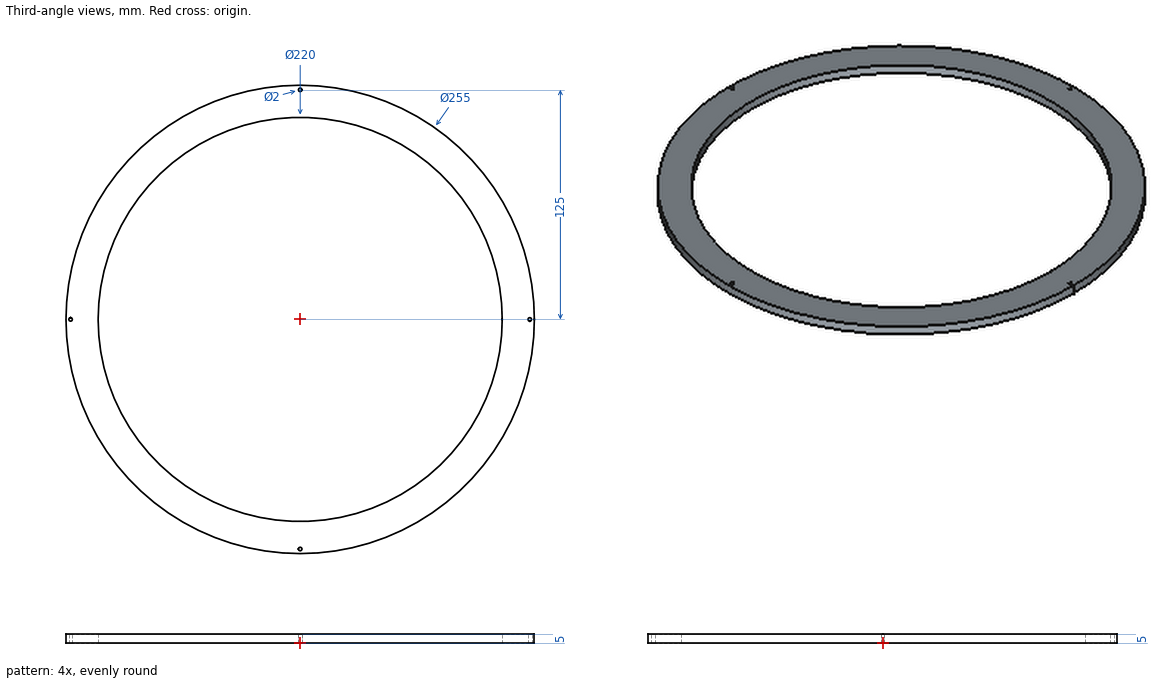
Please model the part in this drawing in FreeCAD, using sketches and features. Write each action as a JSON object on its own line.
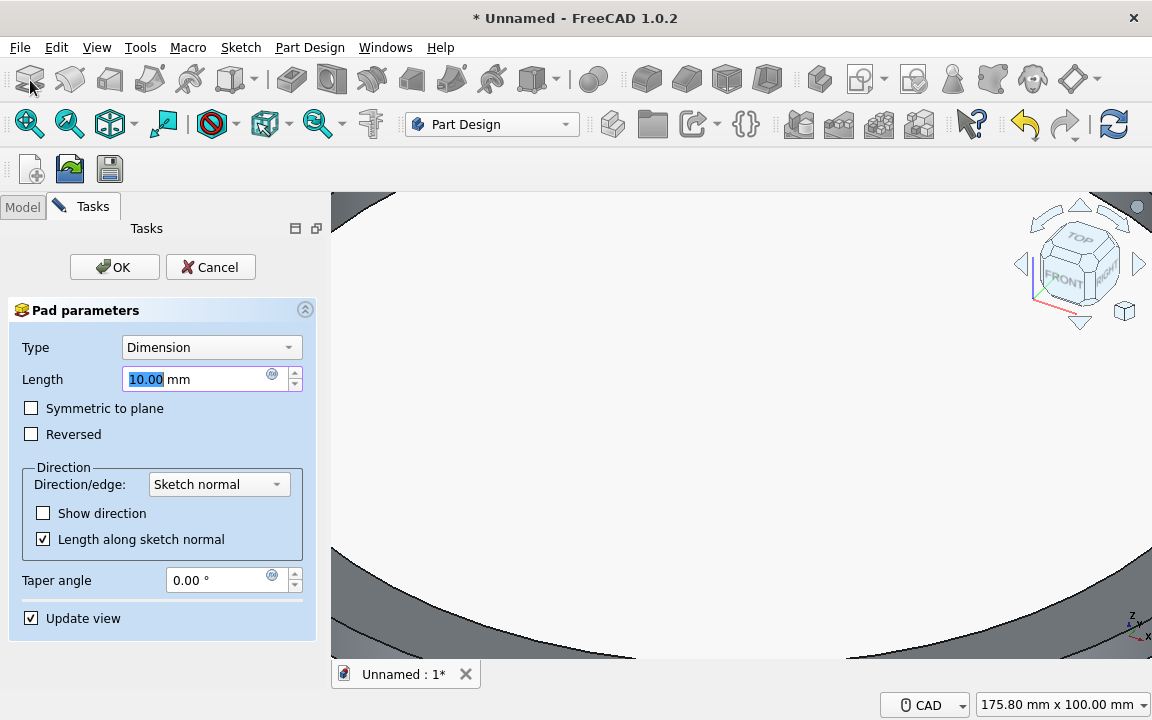
{"action": "type", "text": "5"}
{"action": "key", "text": "Tab"}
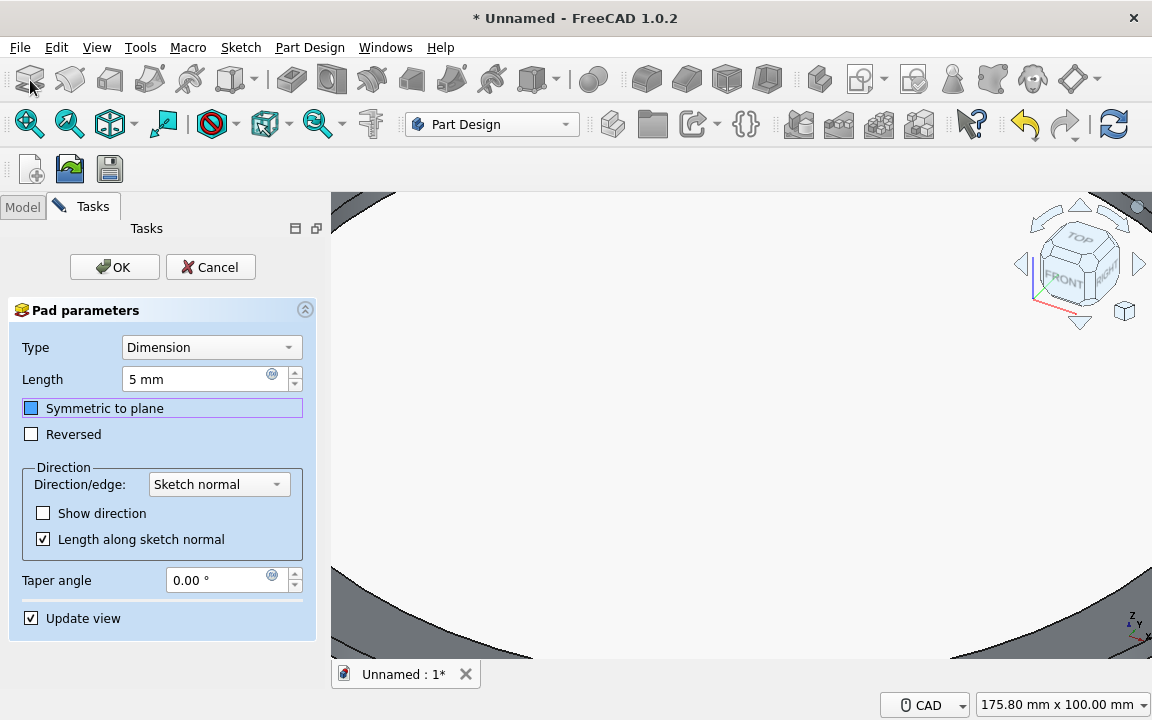
{"action": "left_click", "coordinate": [115, 267]}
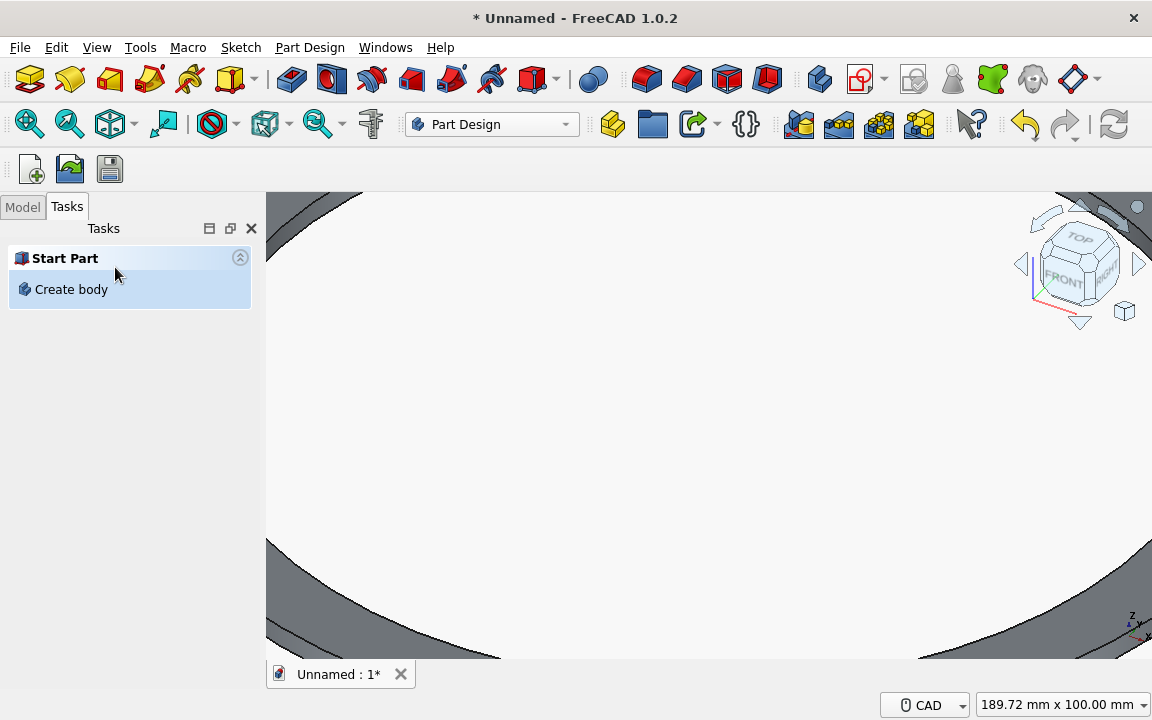
{"action": "left_click", "coordinate": [30, 124]}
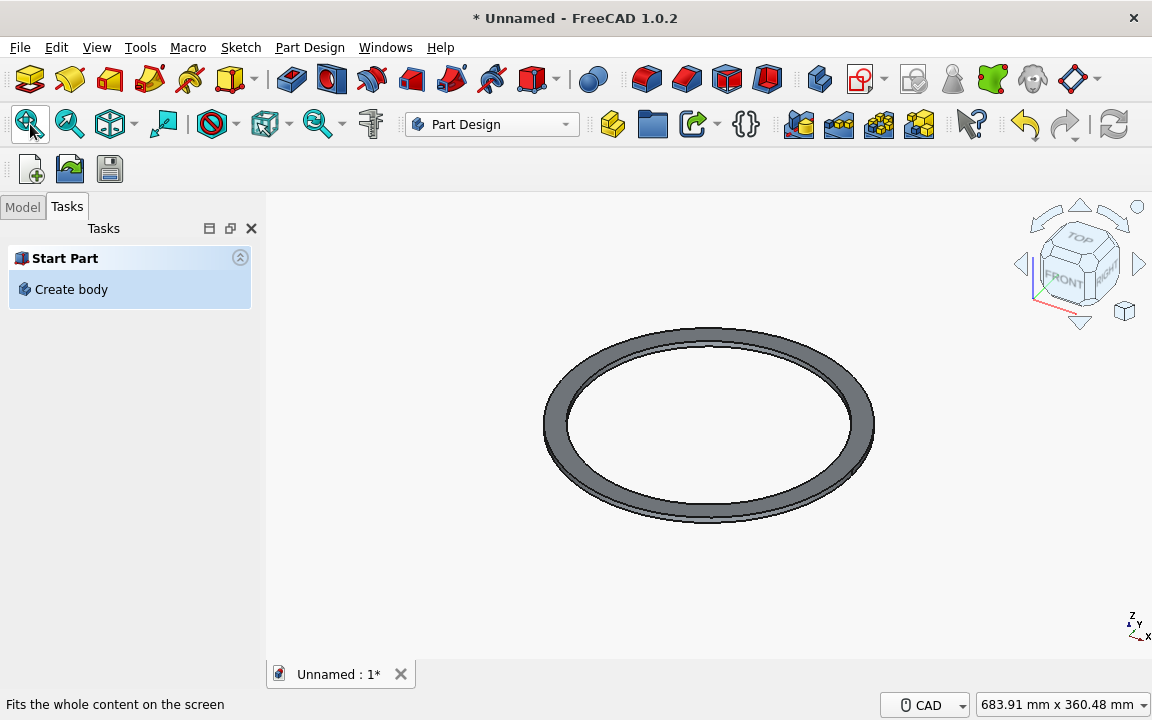
{"action": "left_click", "coordinate": [597, 479]}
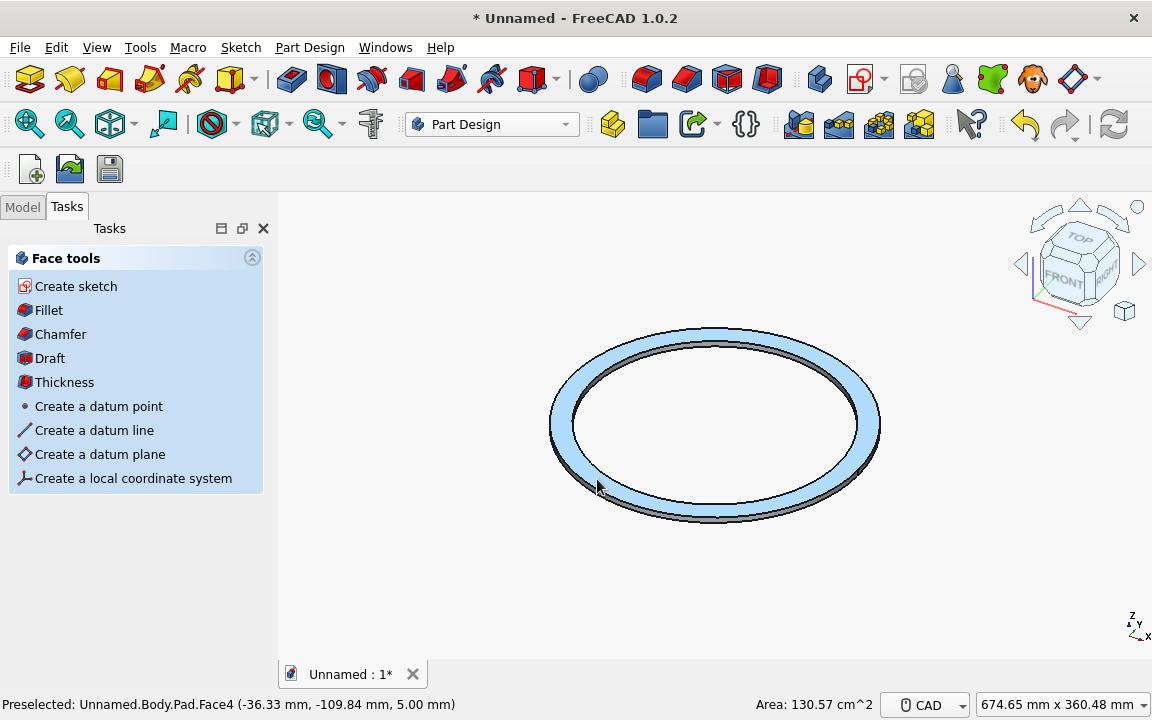
{"action": "left_click", "coordinate": [860, 80]}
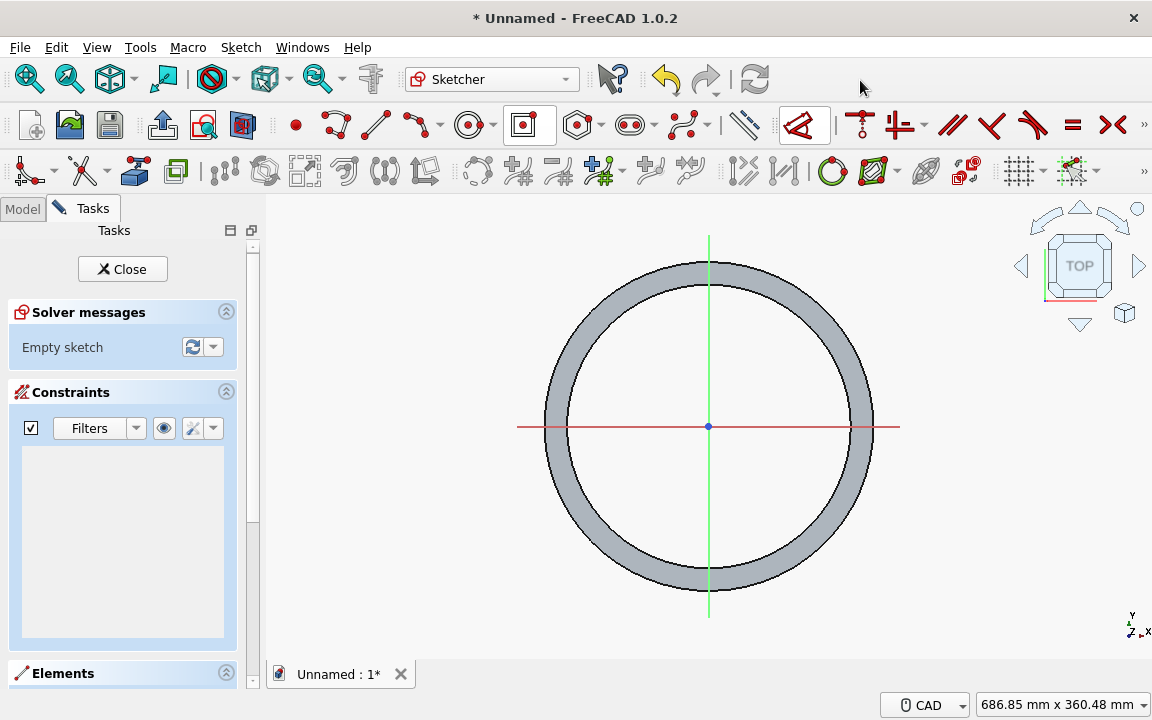
{"action": "scroll", "coordinate": [712, 257], "scroll_direction": "up", "scroll_amount": 15}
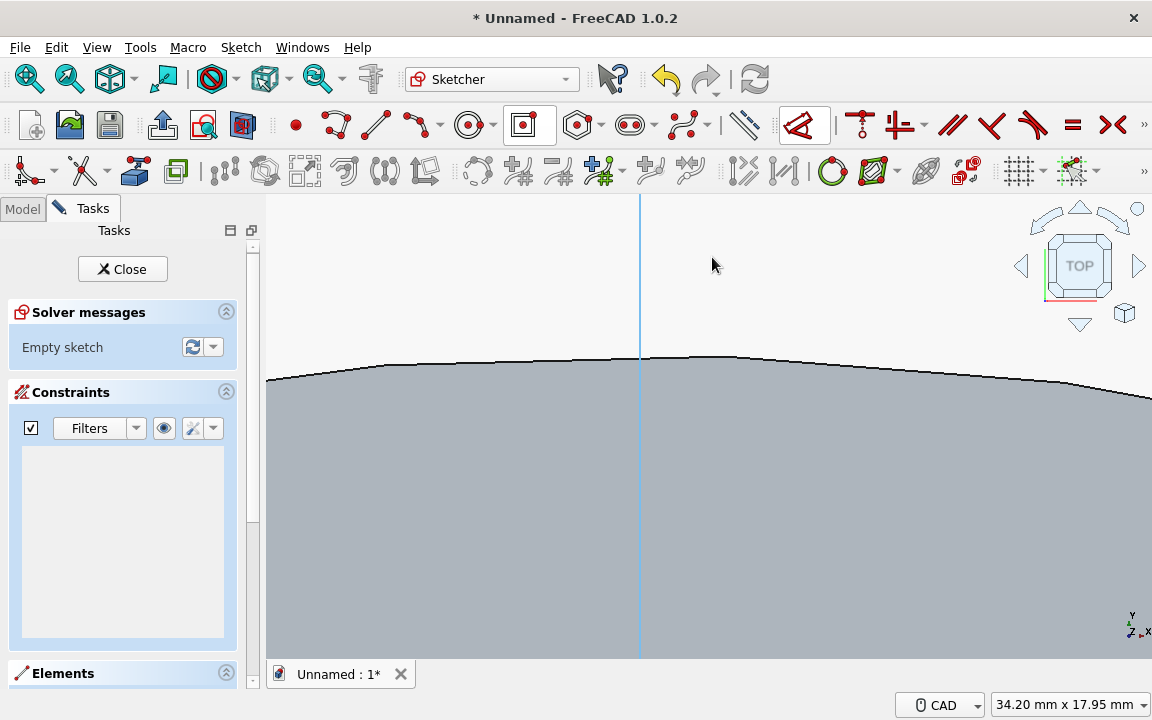
{"action": "scroll", "coordinate": [640, 419], "scroll_direction": "up", "scroll_amount": 9}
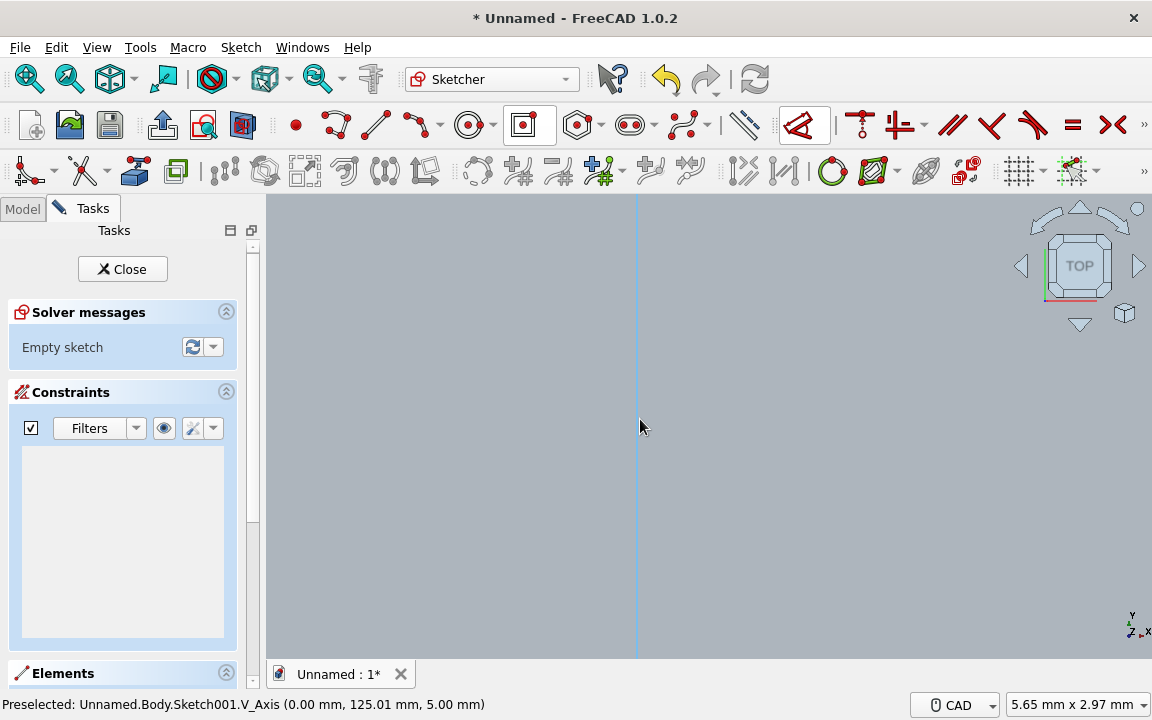
{"action": "left_click", "coordinate": [470, 126]}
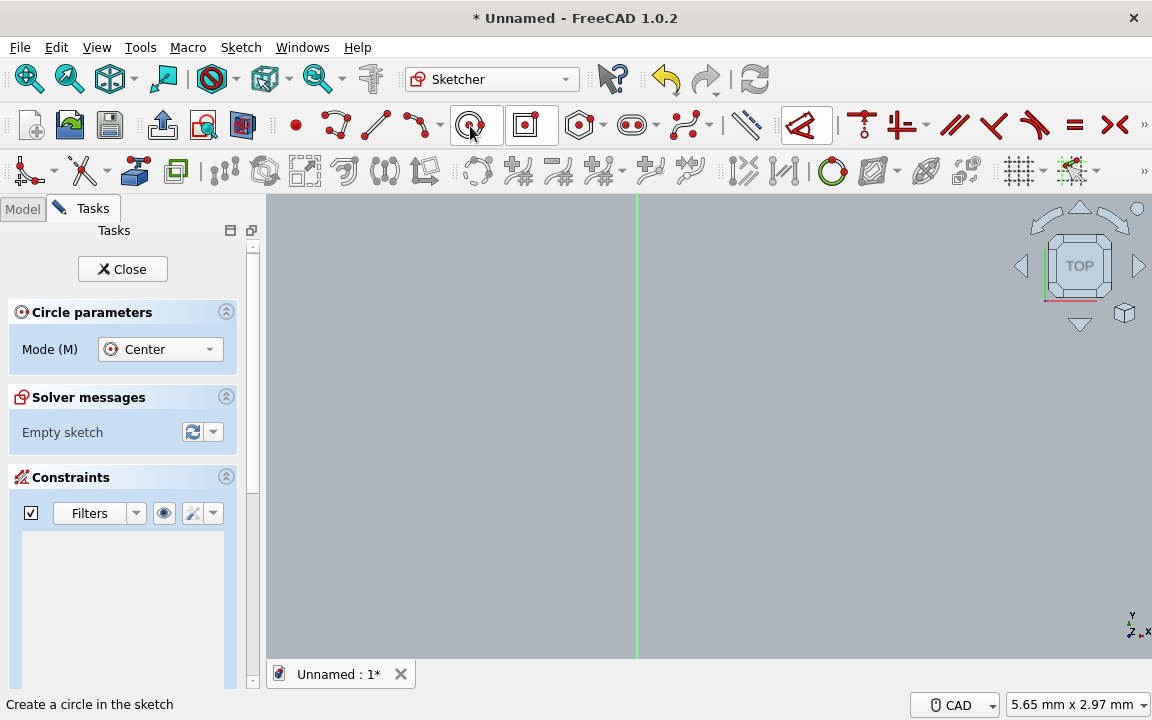
{"action": "left_click", "coordinate": [637, 424]}
{"action": "mouse_move", "coordinate": [748, 313]}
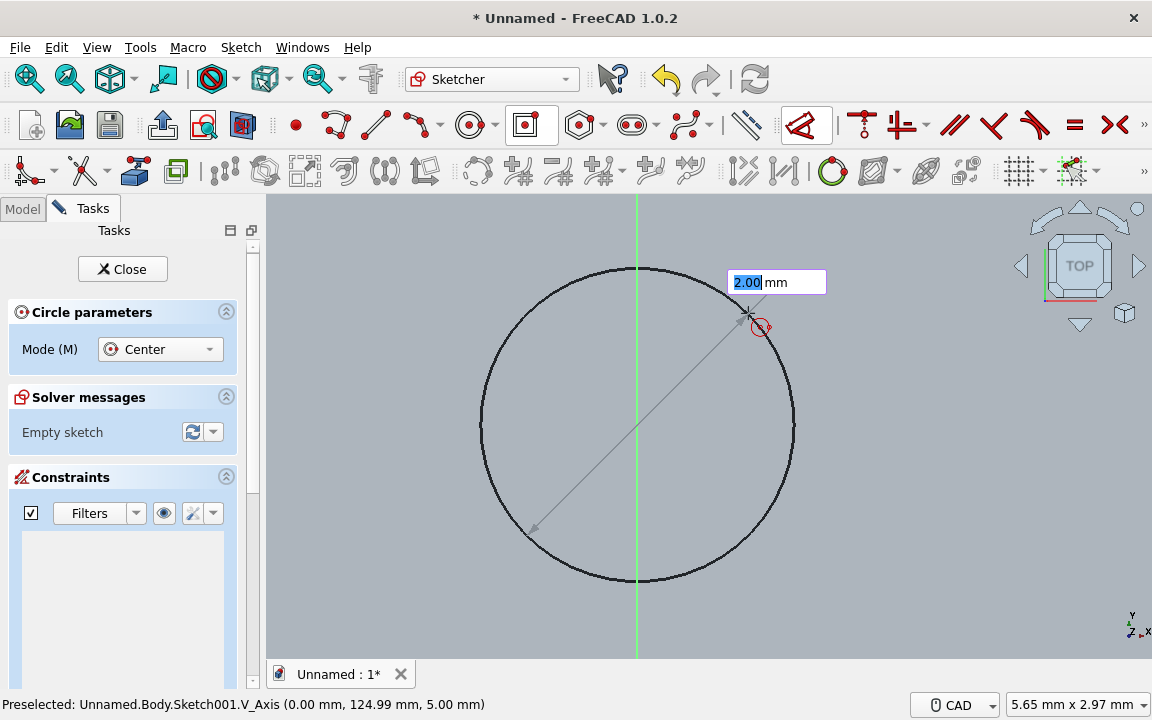
{"action": "type", "text": "2"}
{"action": "key", "text": "Return"}
{"action": "key", "text": "Escape"}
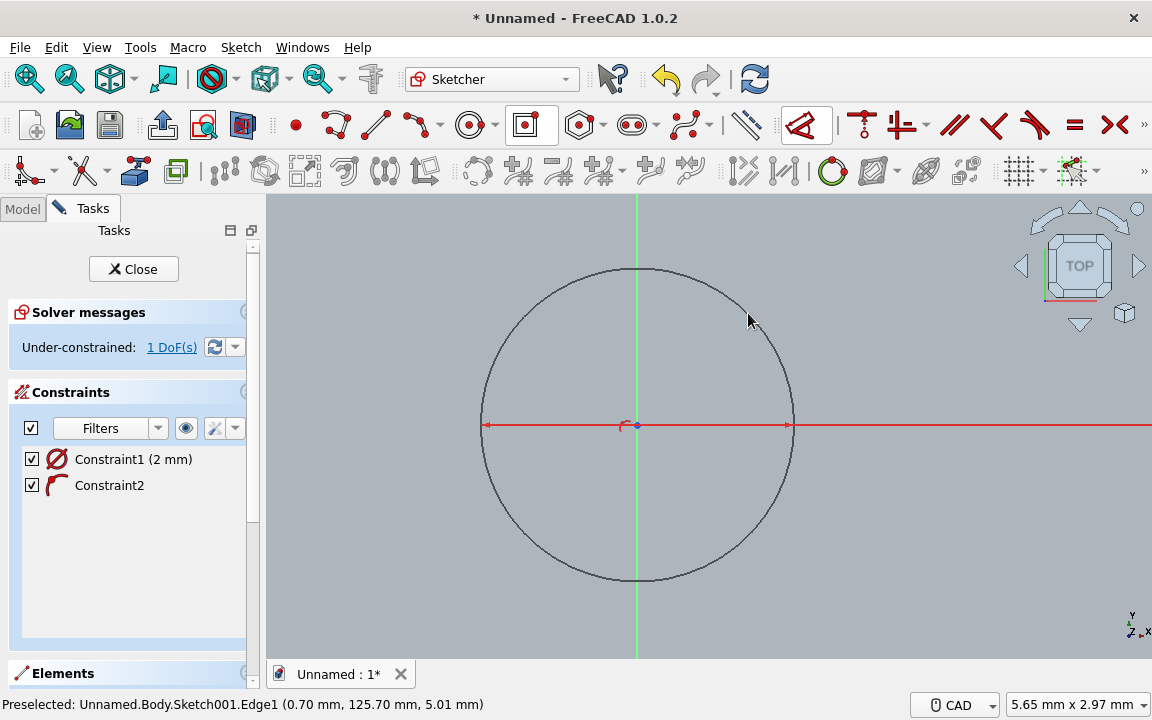
{"action": "left_click", "coordinate": [637, 425]}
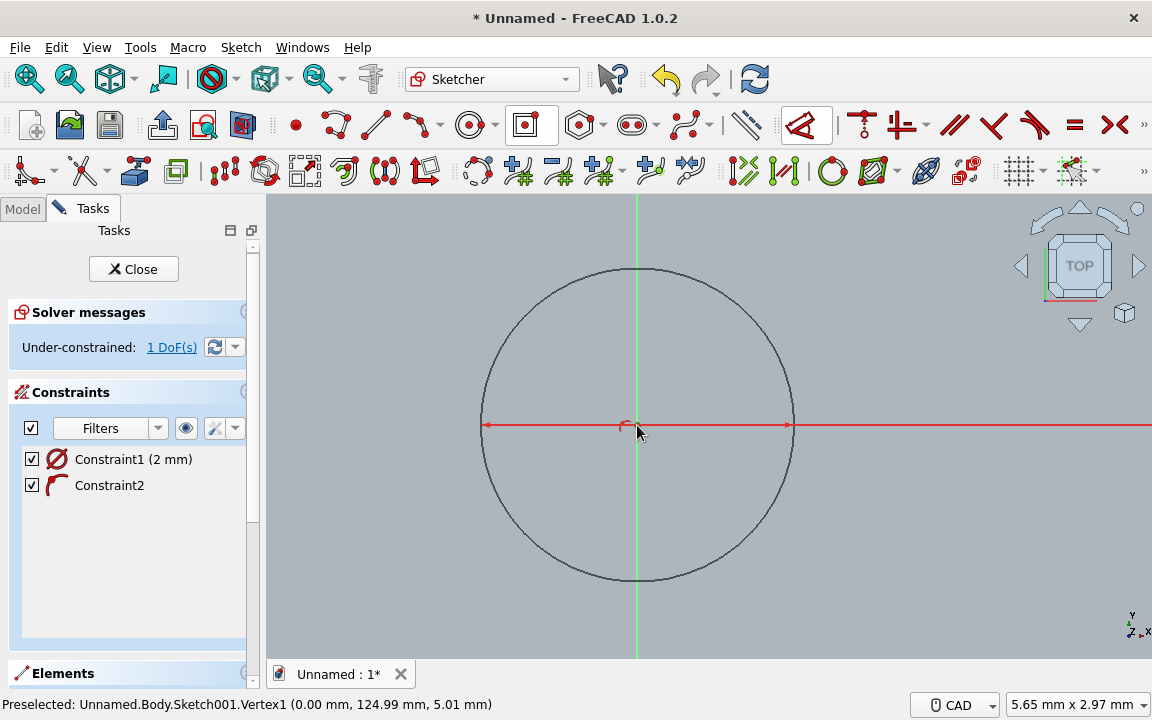
{"action": "key", "text": "i"}